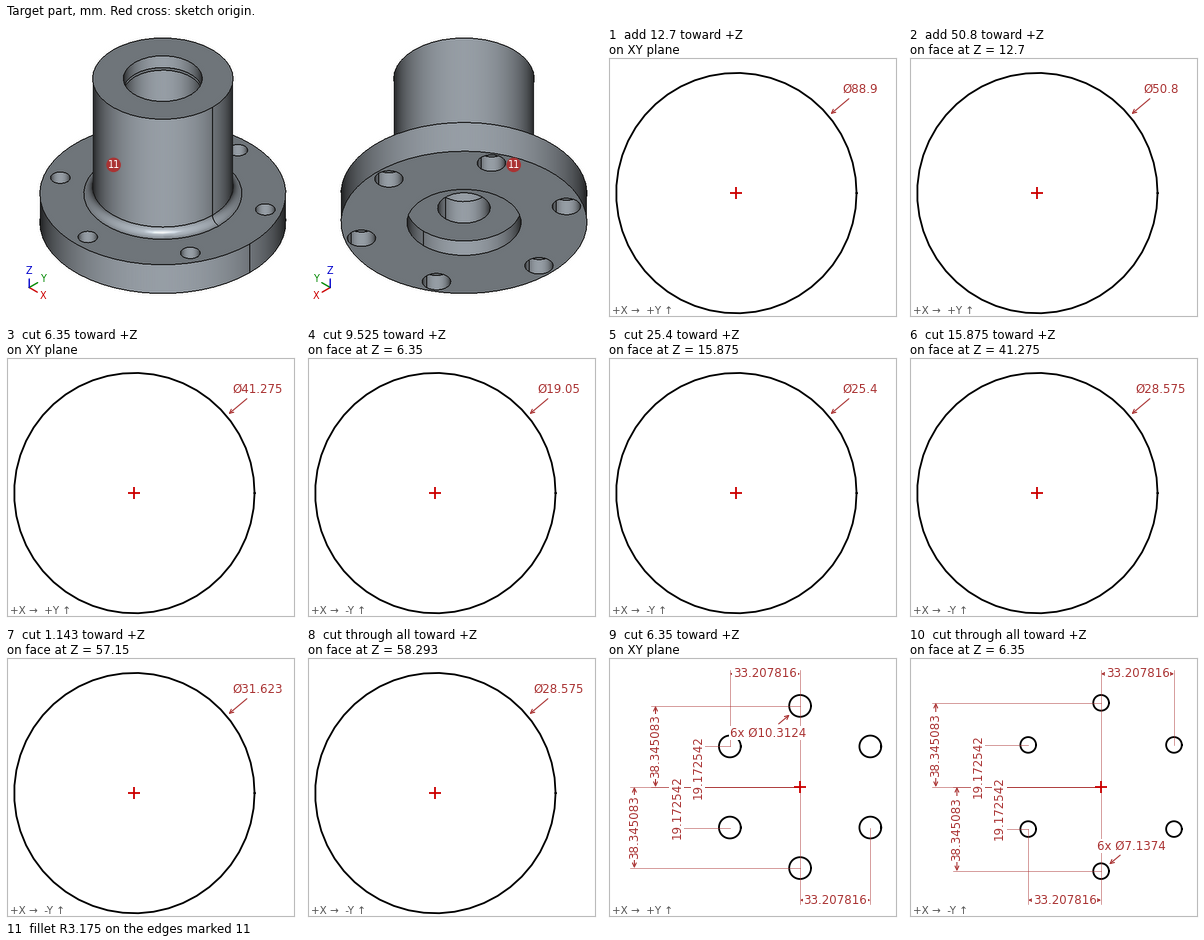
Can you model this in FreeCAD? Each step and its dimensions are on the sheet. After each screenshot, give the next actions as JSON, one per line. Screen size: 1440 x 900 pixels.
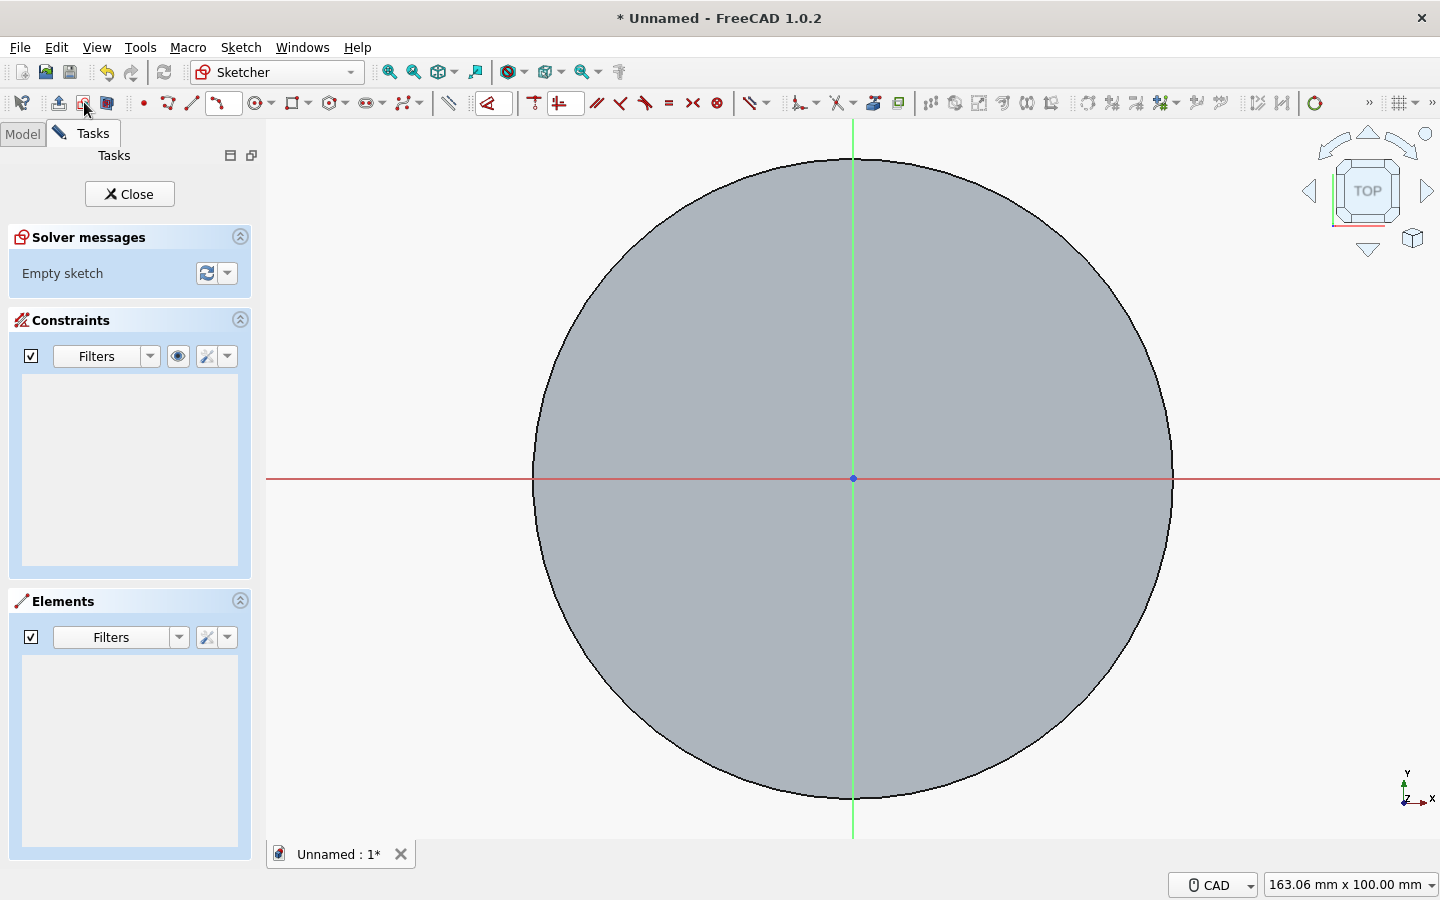
{"action": "left_click", "coordinate": [256, 104]}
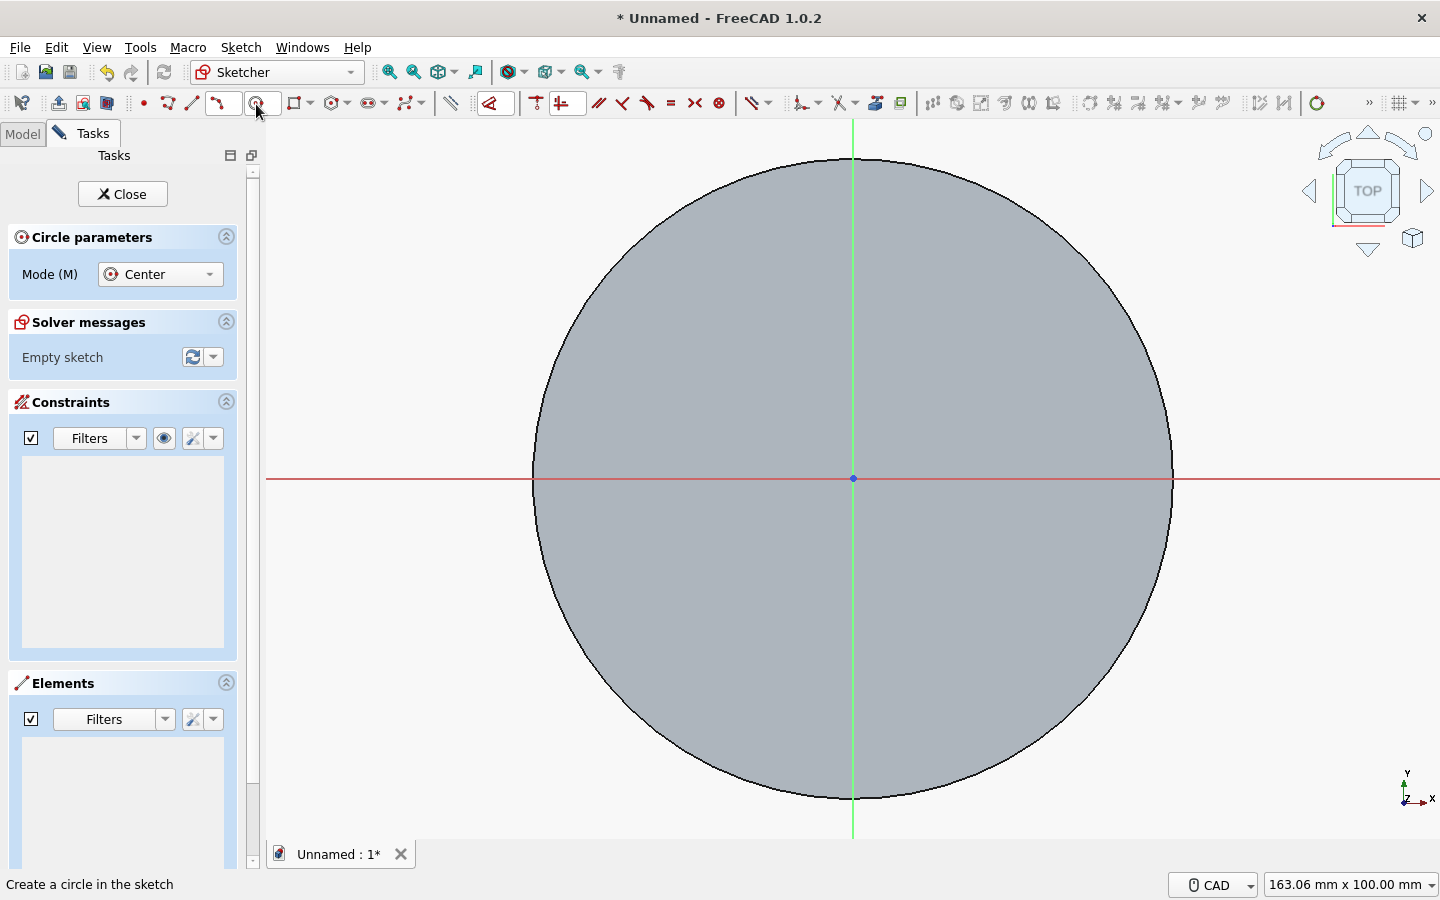
{"action": "left_click", "coordinate": [853, 479]}
{"action": "mouse_move", "coordinate": [982, 350]}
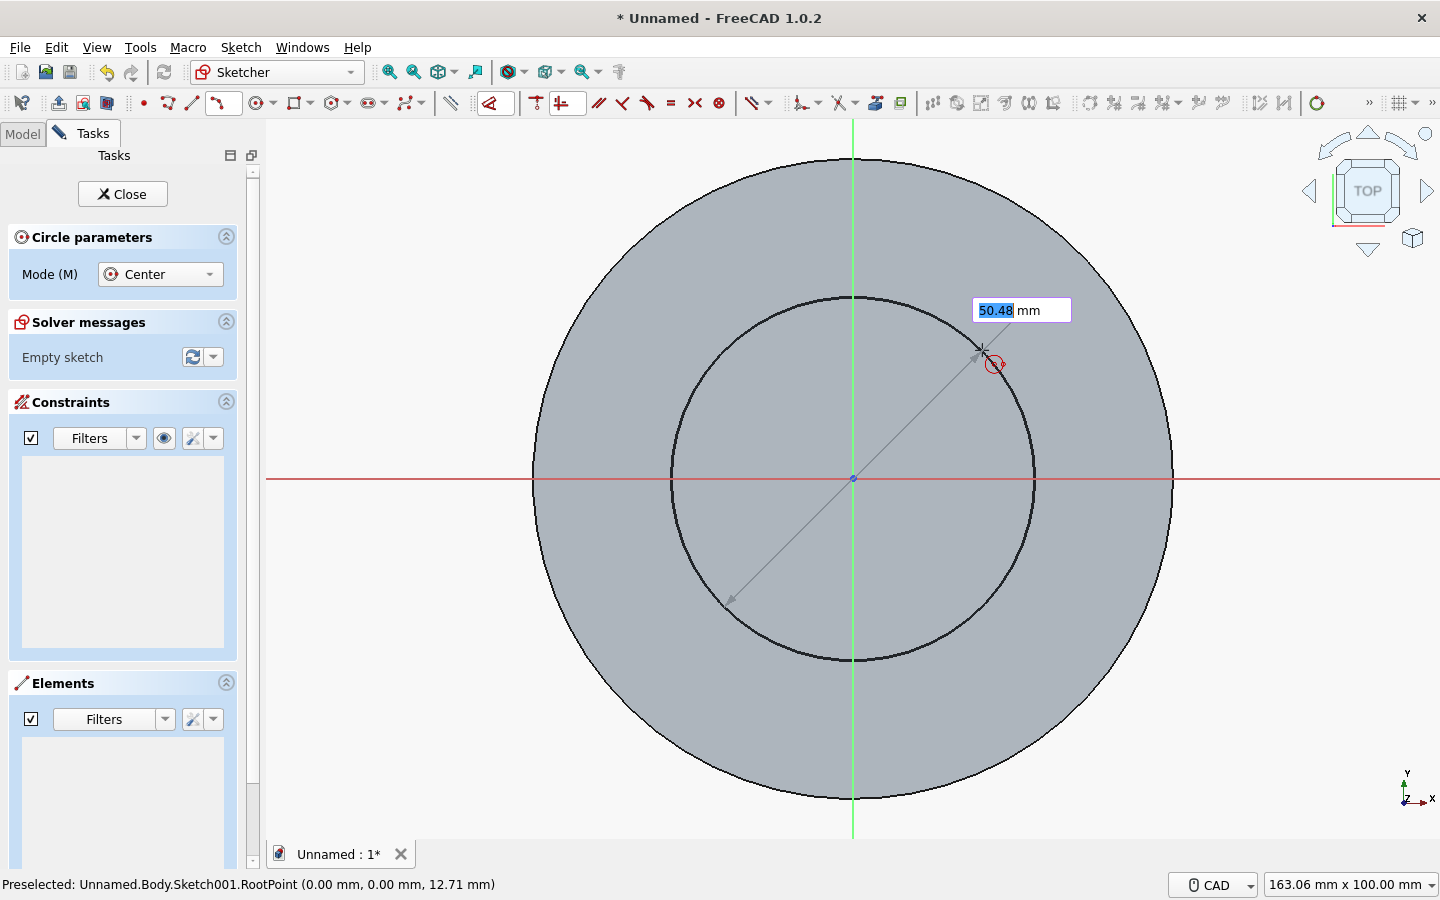
{"action": "type", "text": "50.8"}
{"action": "key", "text": "Return"}
{"action": "key", "text": "Escape"}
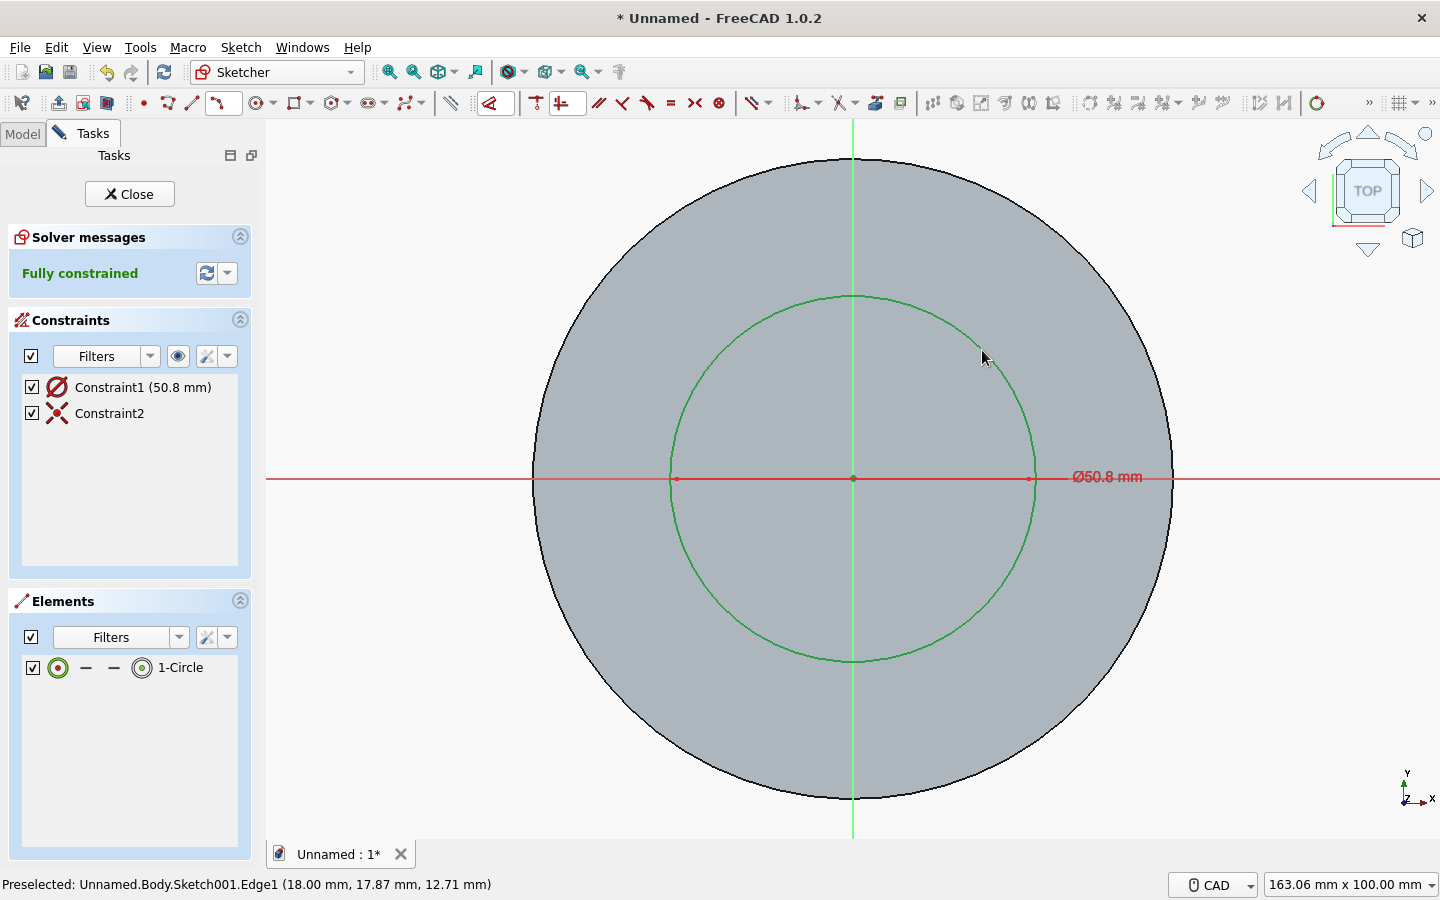
{"action": "left_click", "coordinate": [130, 194]}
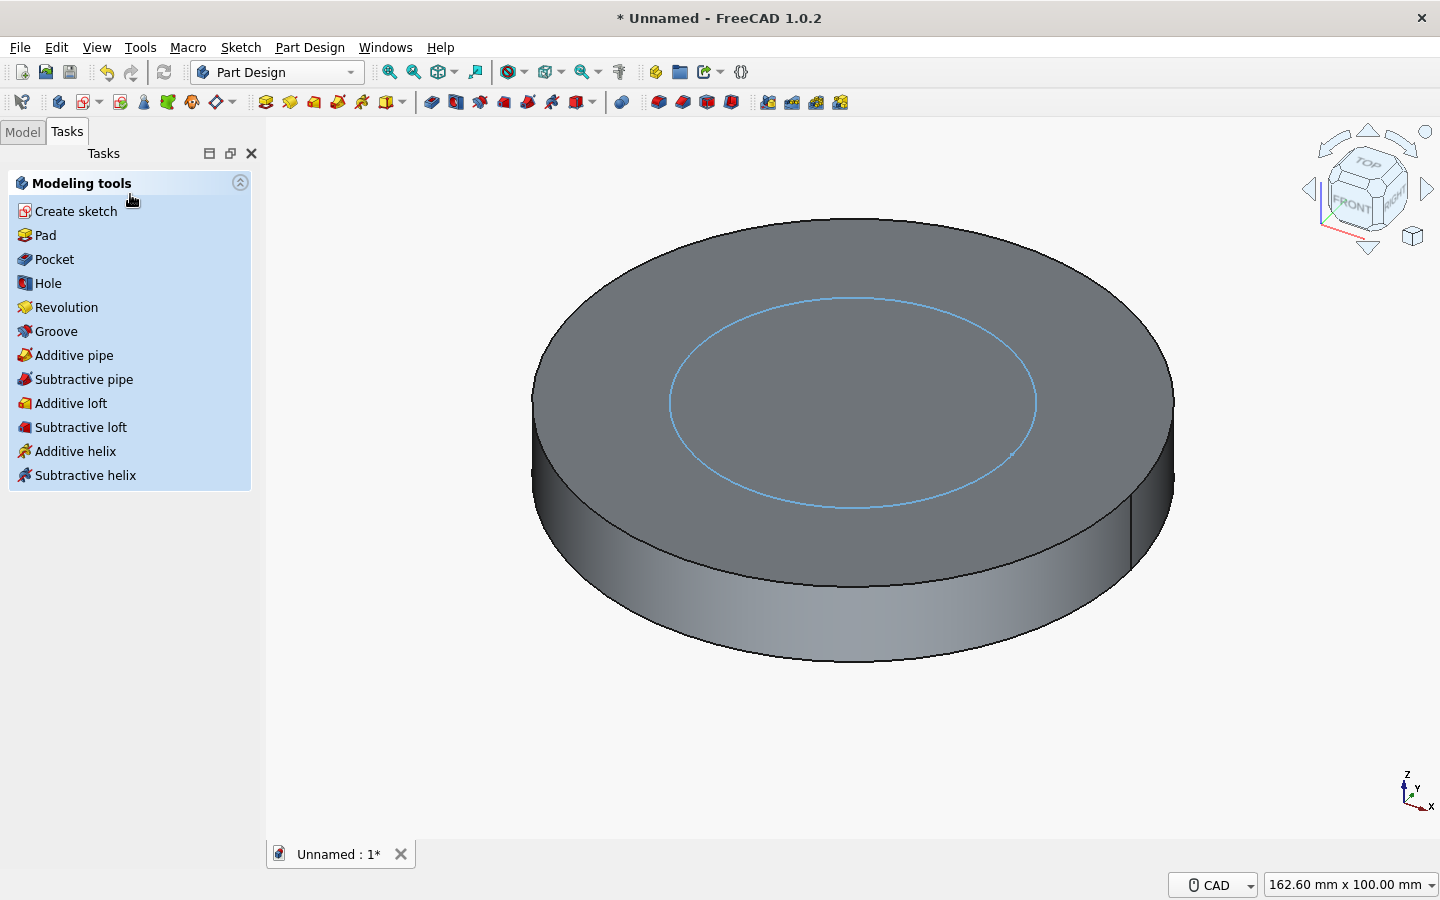
{"action": "left_click", "coordinate": [266, 102]}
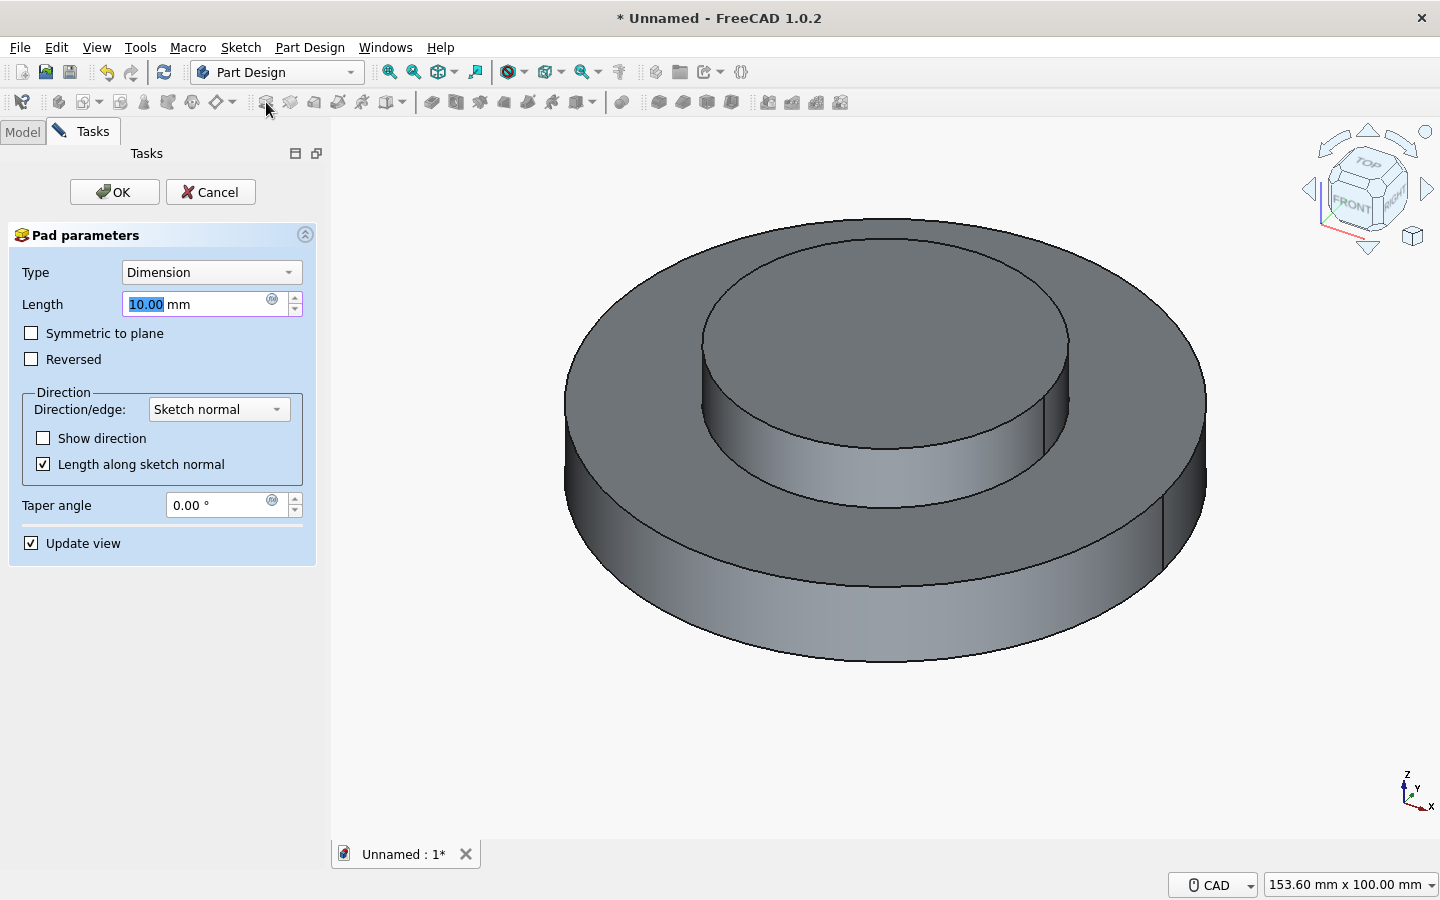
{"action": "type", "text": "50.8"}
{"action": "key", "text": "Tab"}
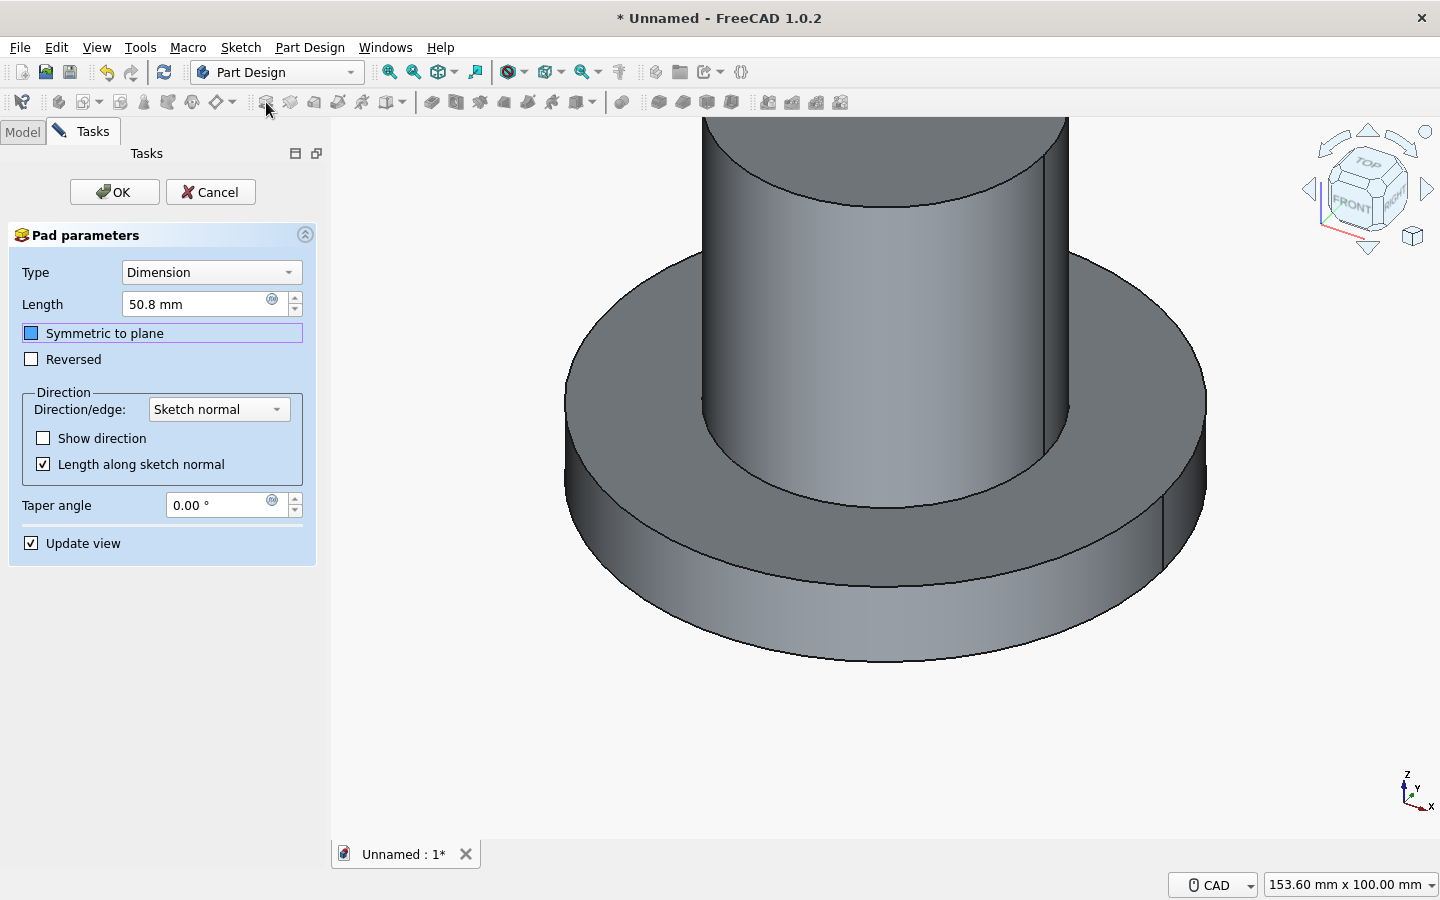
{"action": "left_click", "coordinate": [115, 192]}